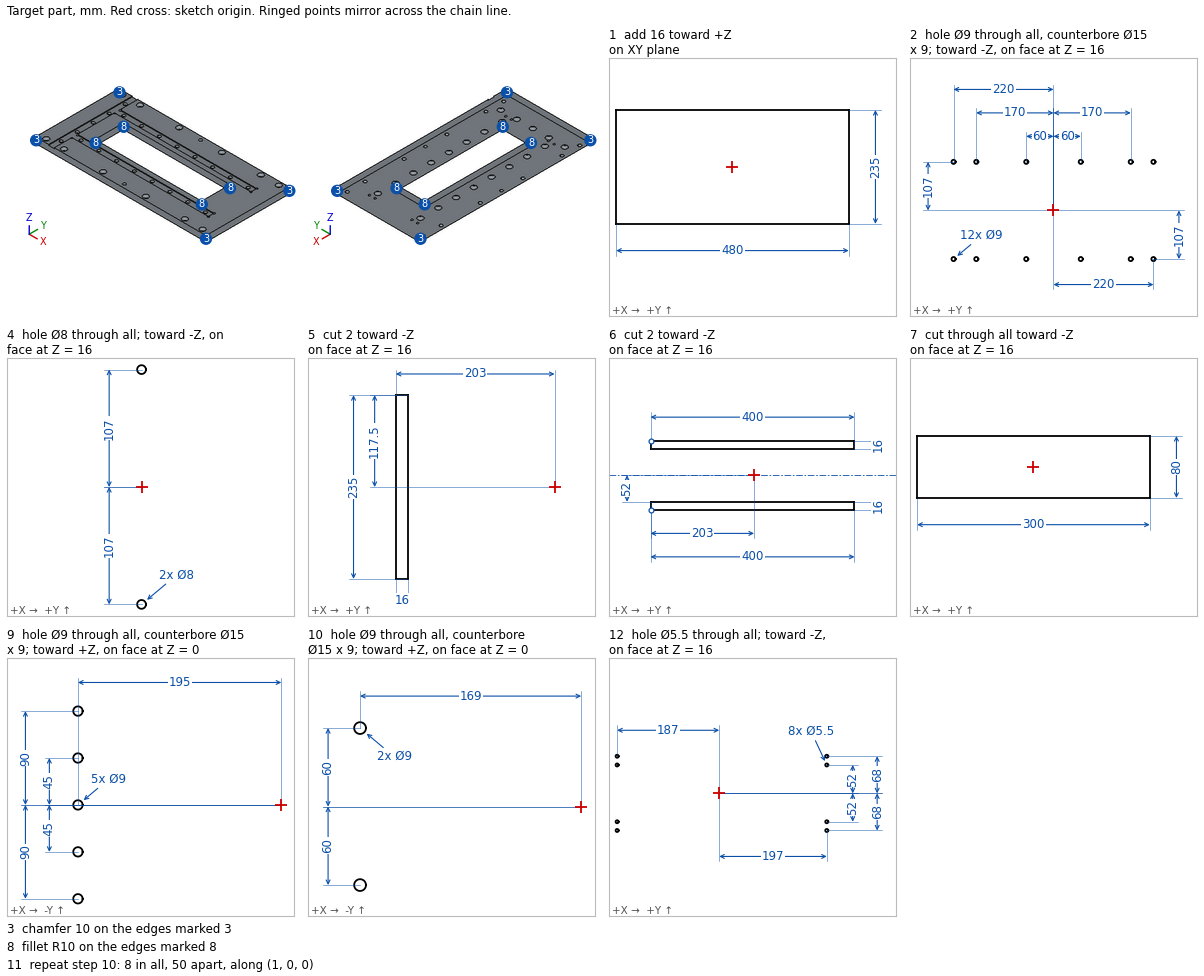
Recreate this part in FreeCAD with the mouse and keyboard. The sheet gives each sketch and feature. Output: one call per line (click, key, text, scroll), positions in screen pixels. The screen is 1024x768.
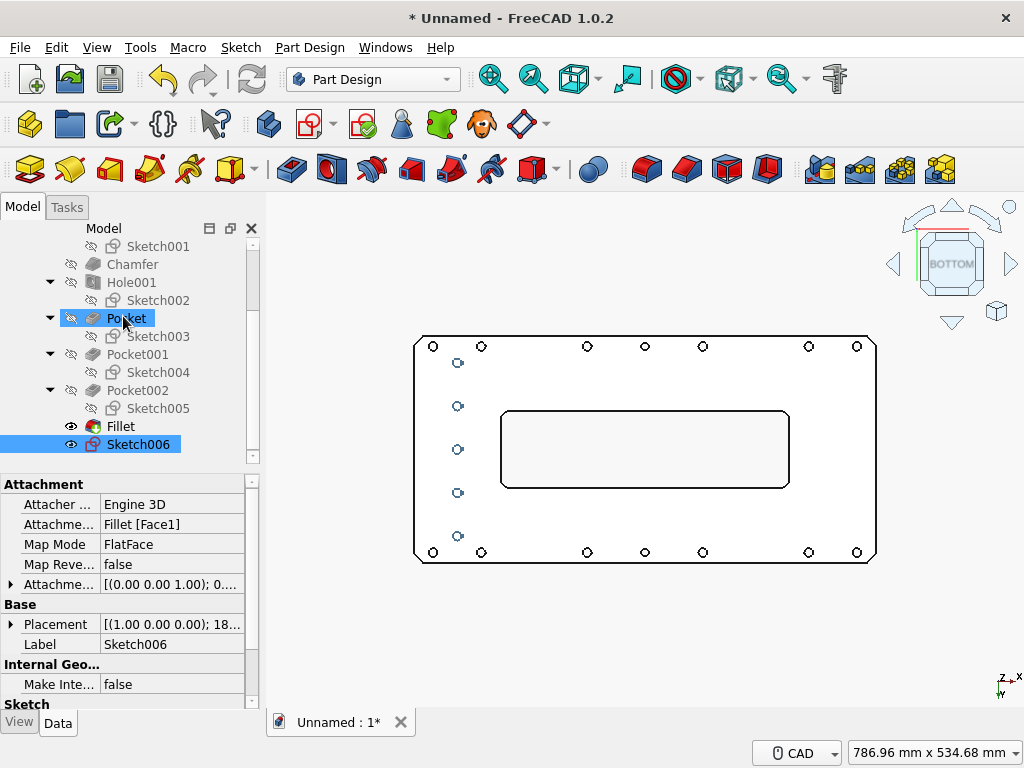
click(332, 170)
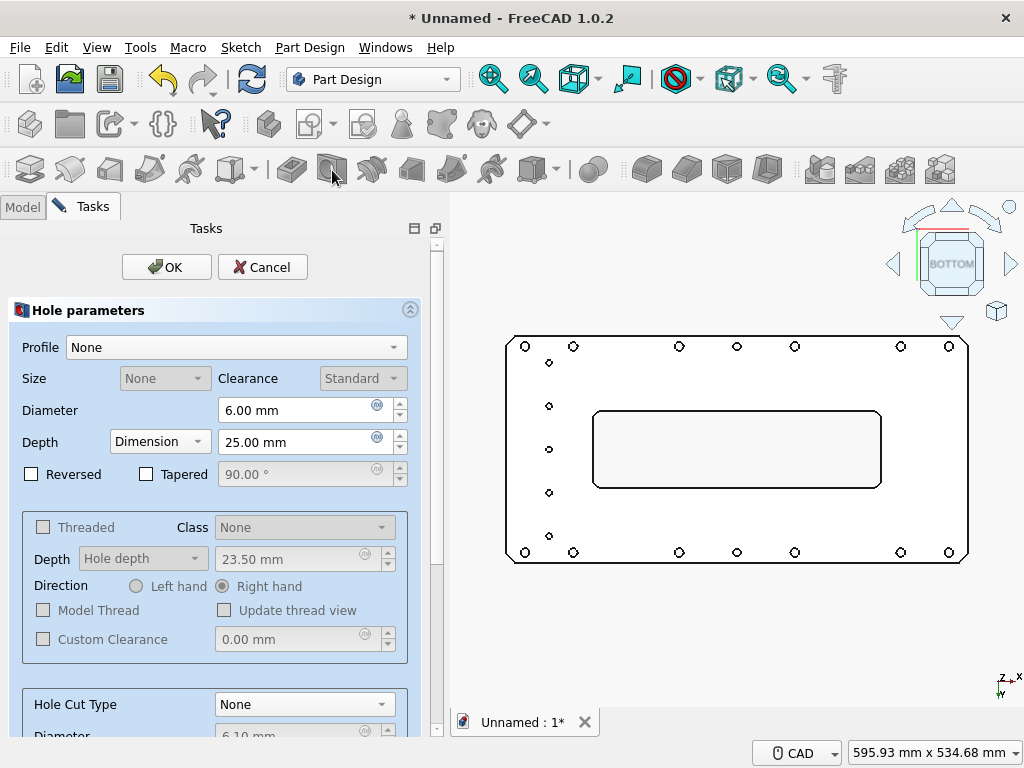
triple_click(305, 410)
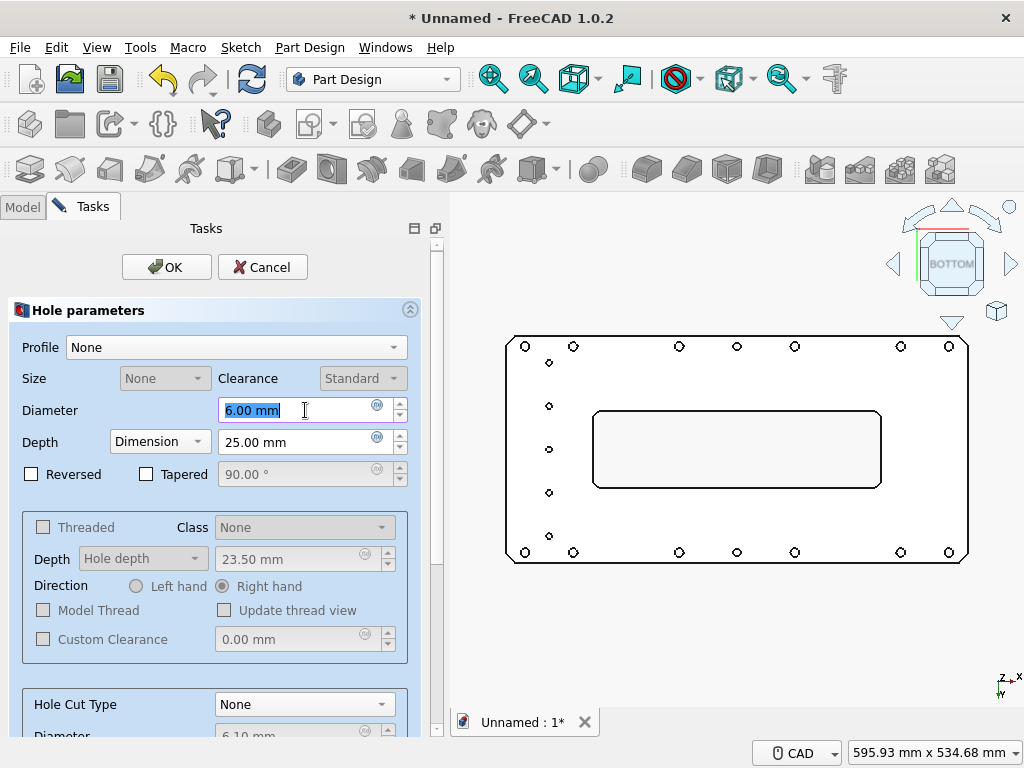
text(9)
key(Tab)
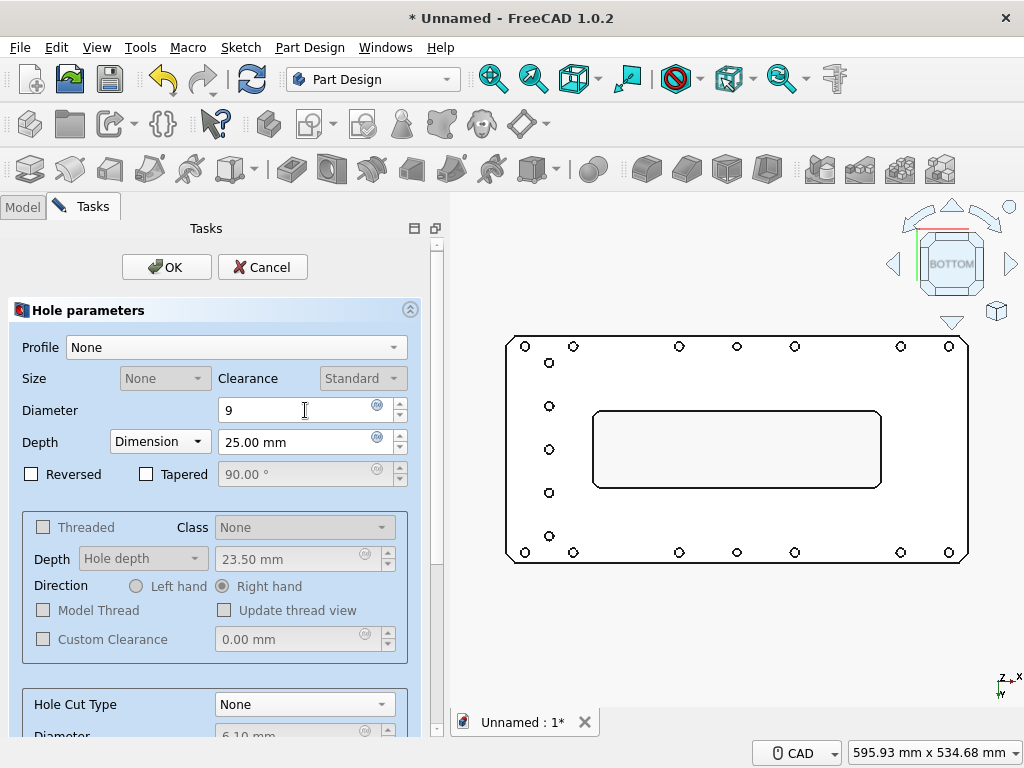
click(161, 442)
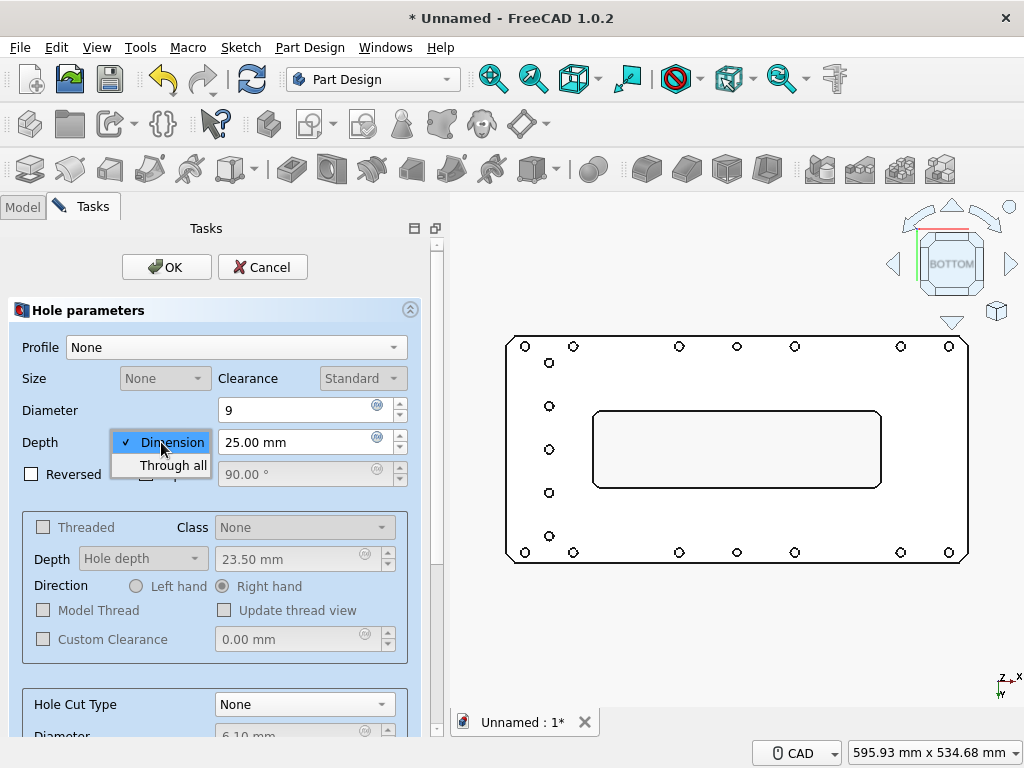
click(160, 466)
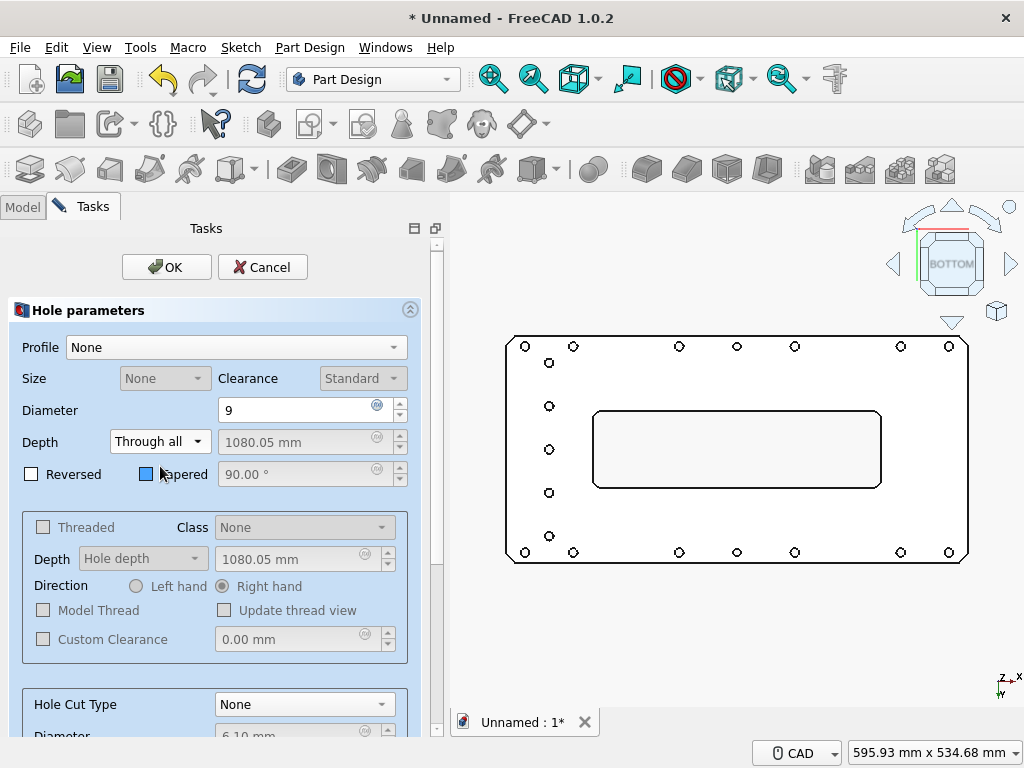
click(306, 704)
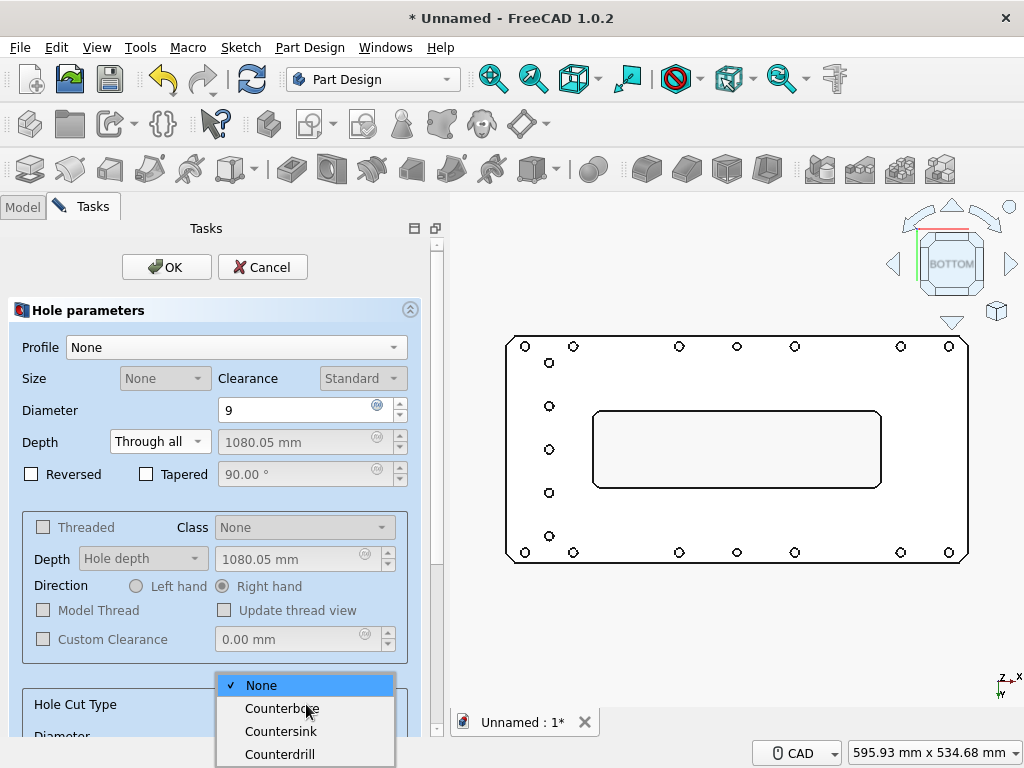
click(304, 708)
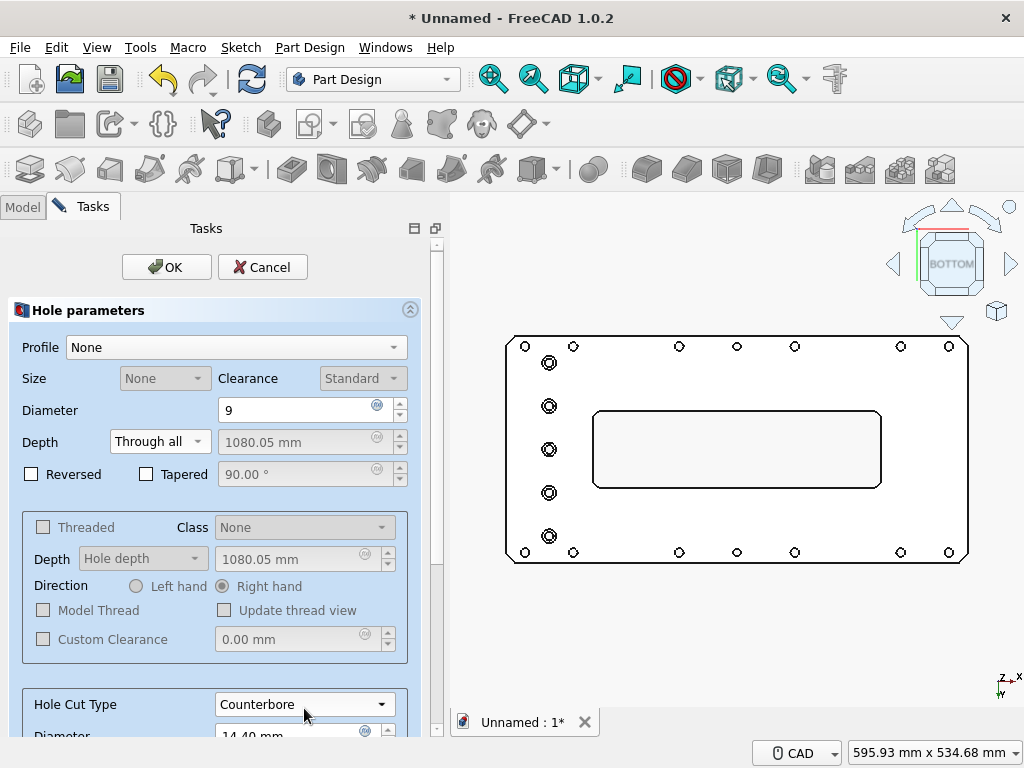
scroll(437, 487, down, 2)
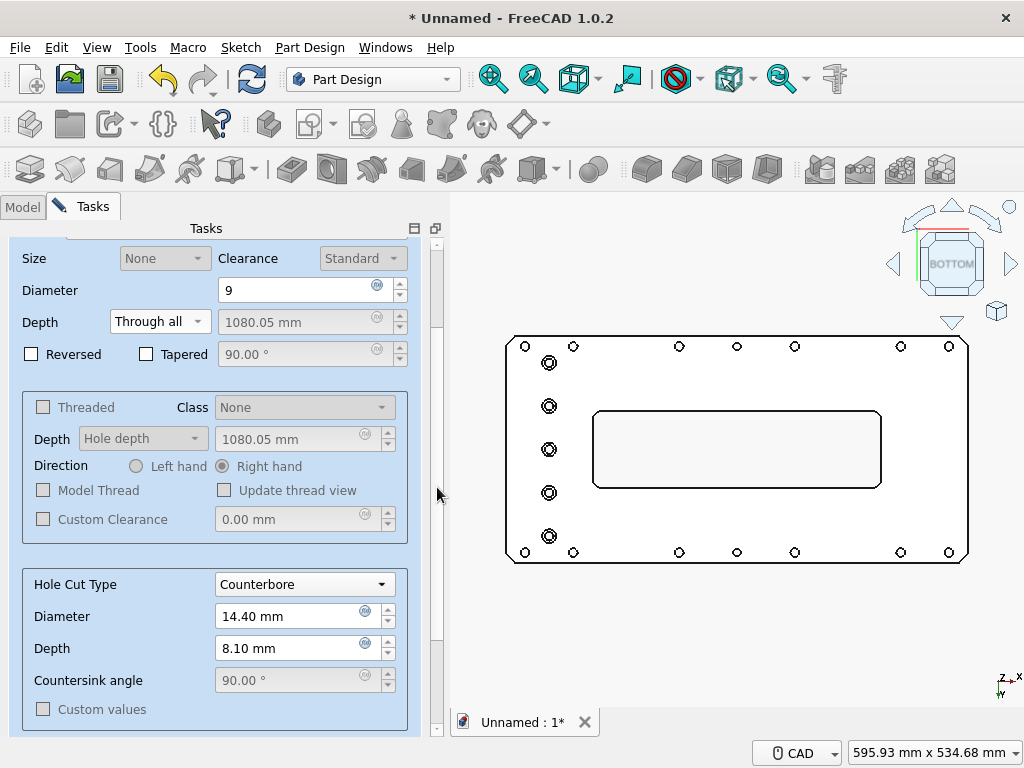
triple_click(298, 616)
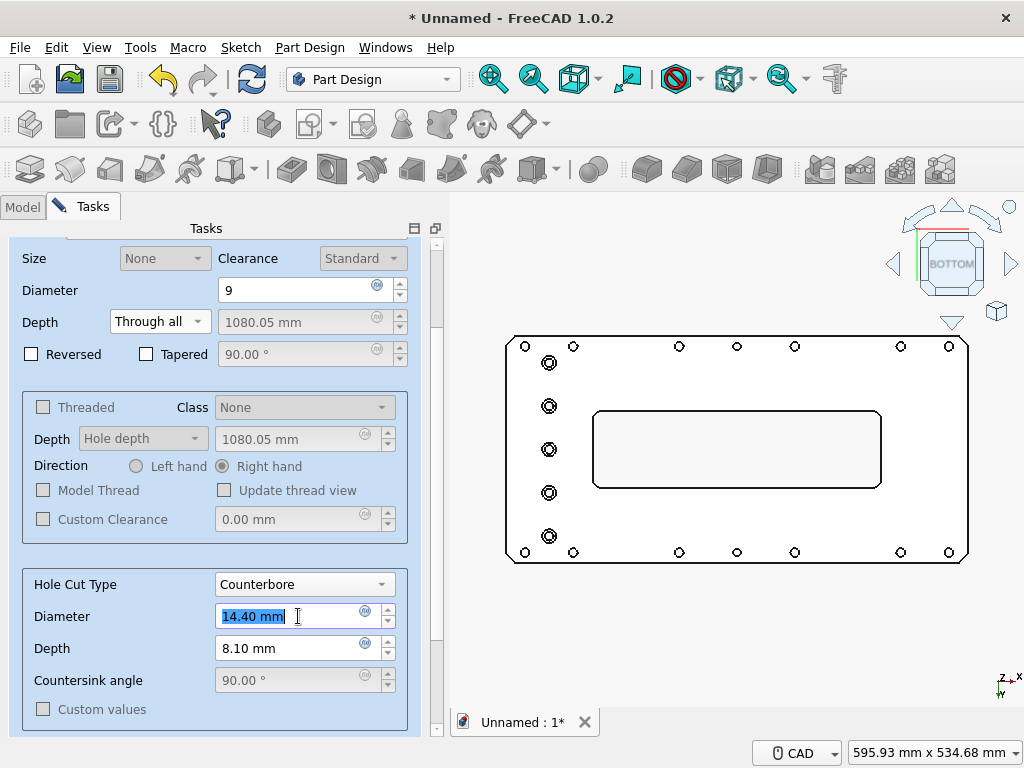
text(15)
key(Tab)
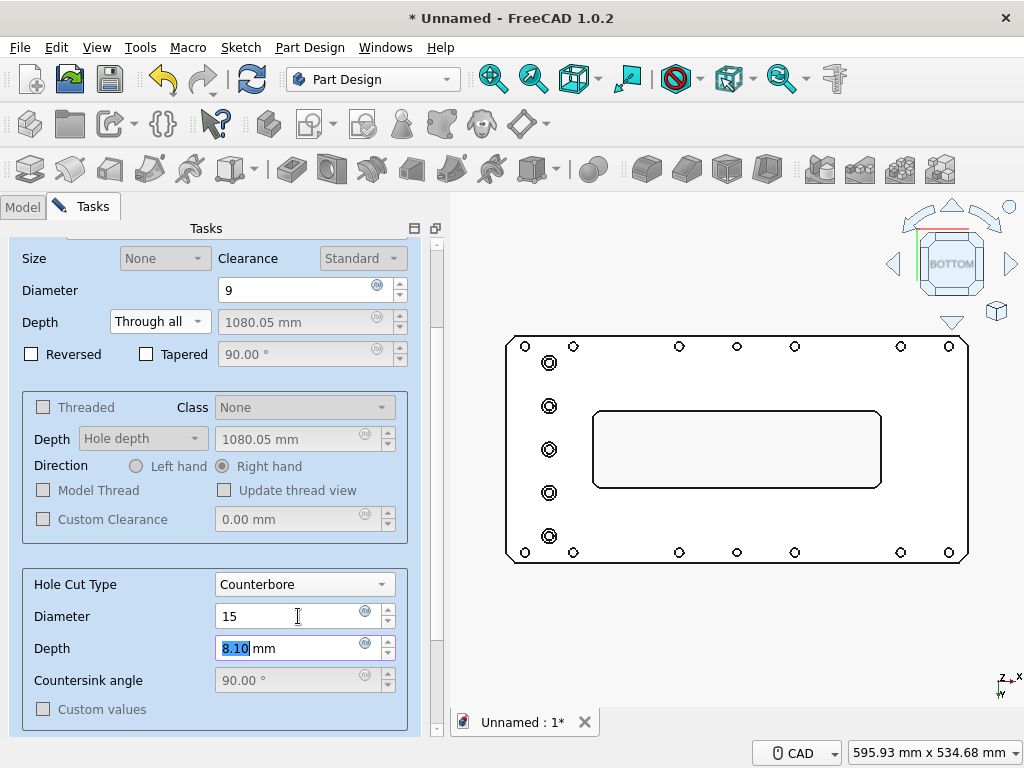
text(9)
key(Tab)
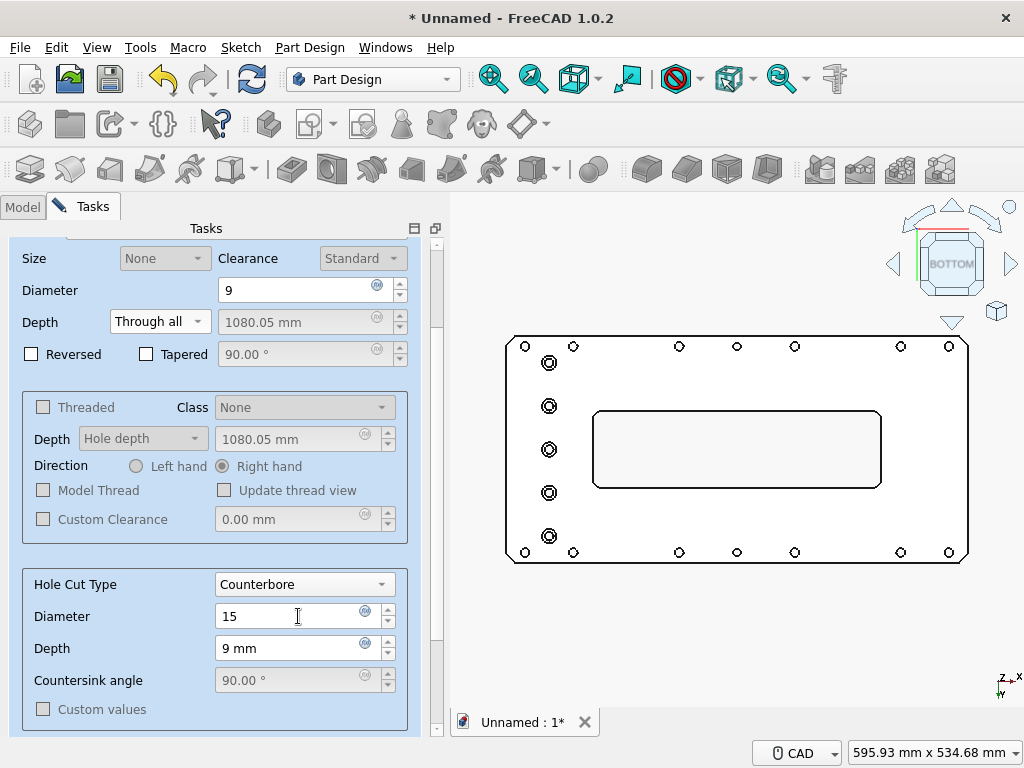
scroll(437, 487, up, 3)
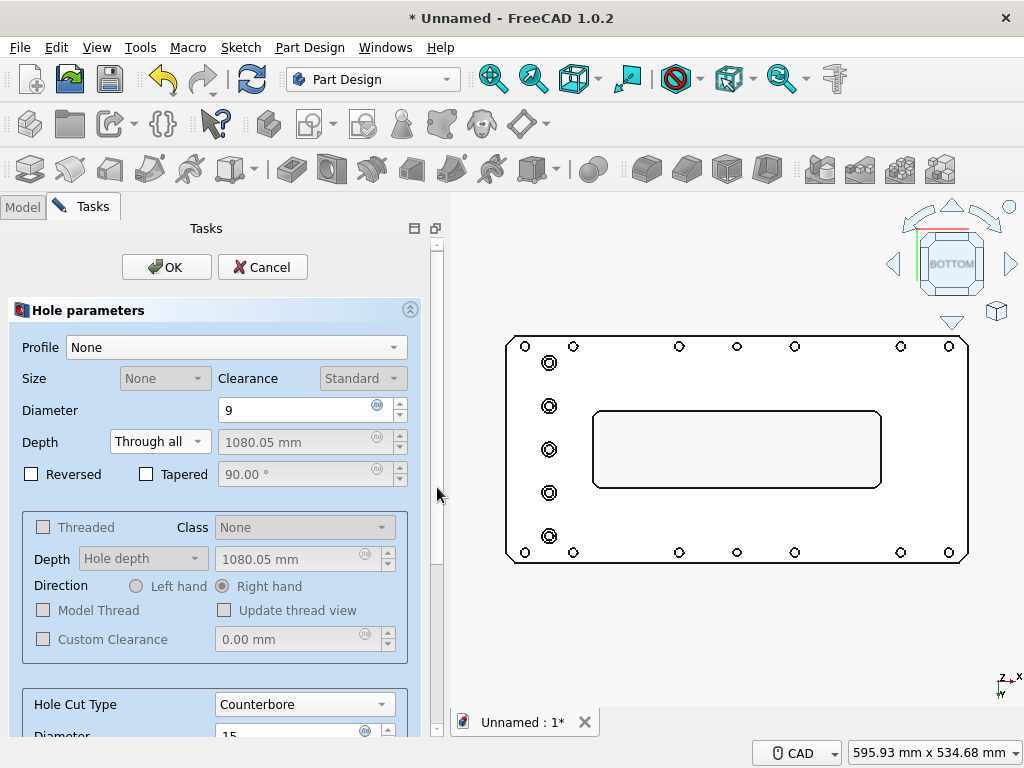
click(167, 267)